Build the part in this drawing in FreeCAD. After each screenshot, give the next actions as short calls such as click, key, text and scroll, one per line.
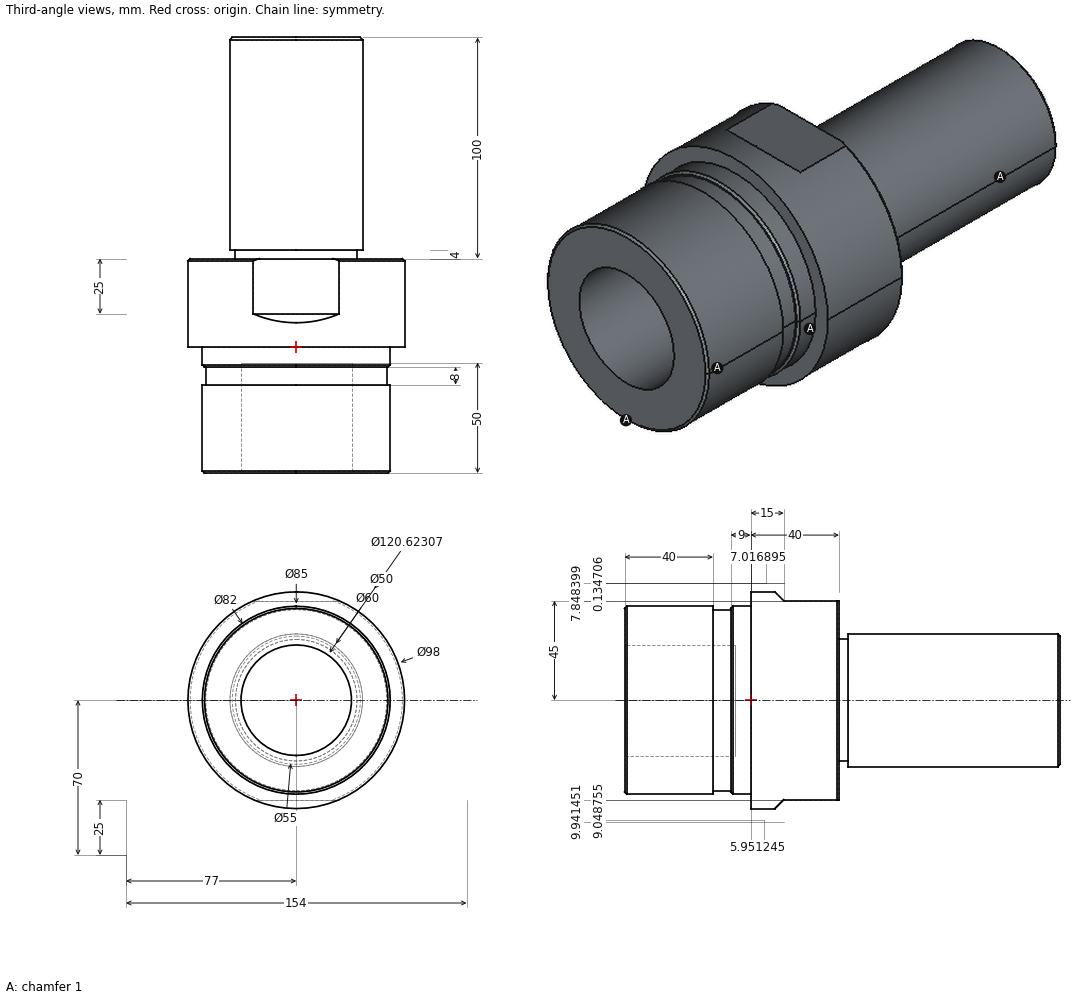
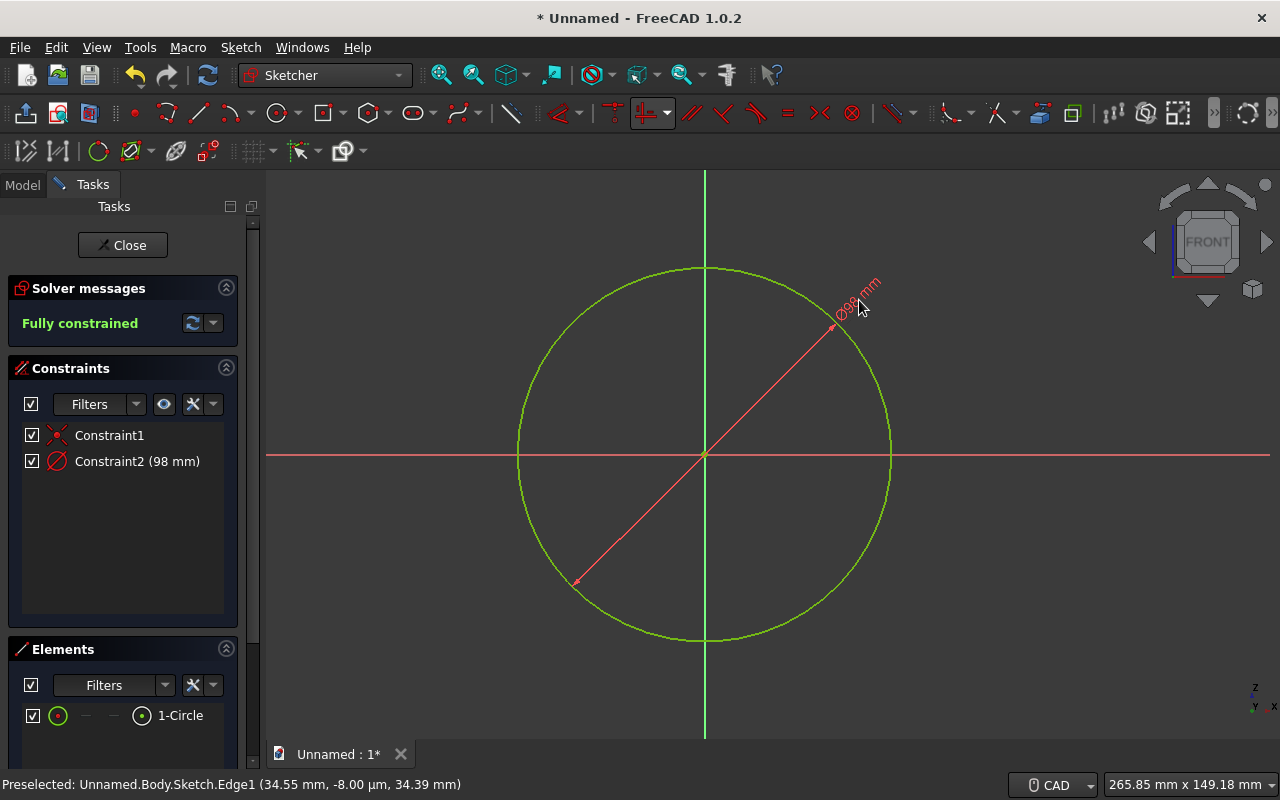
click(123, 245)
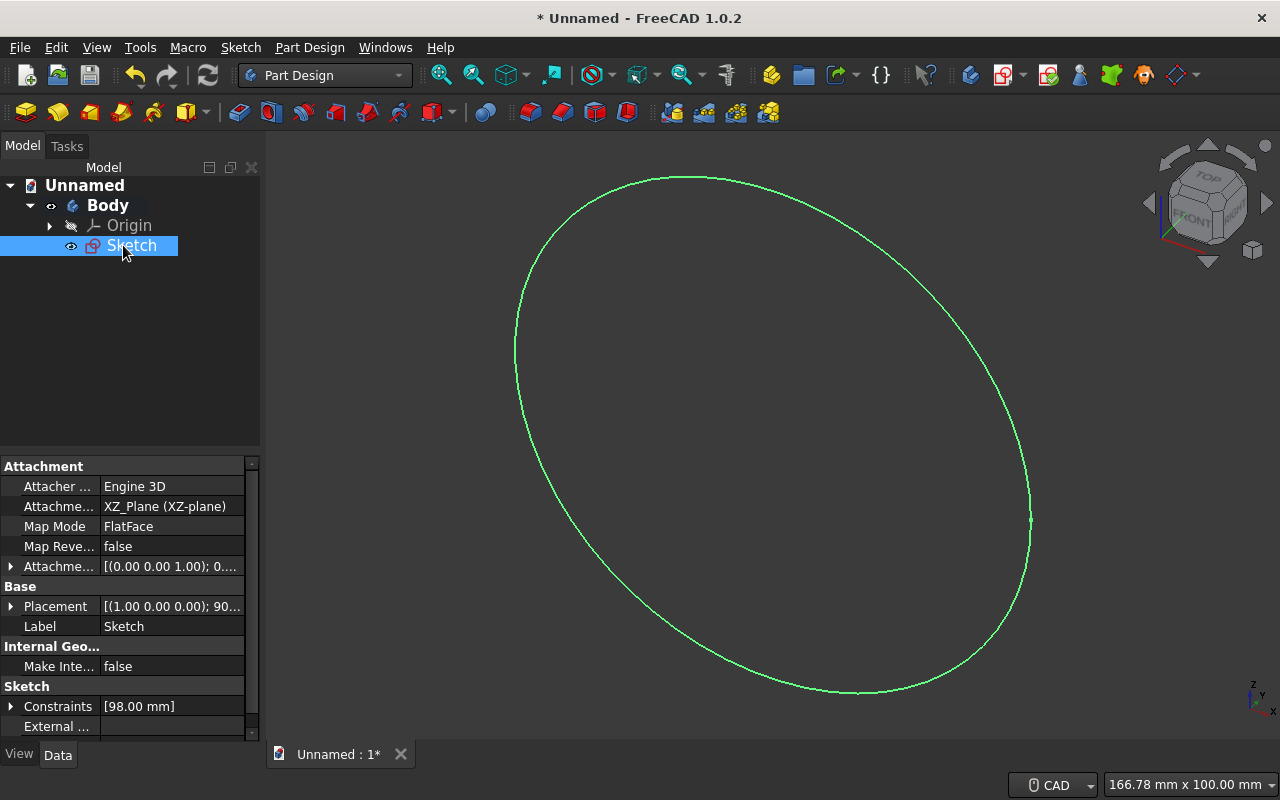
click(26, 112)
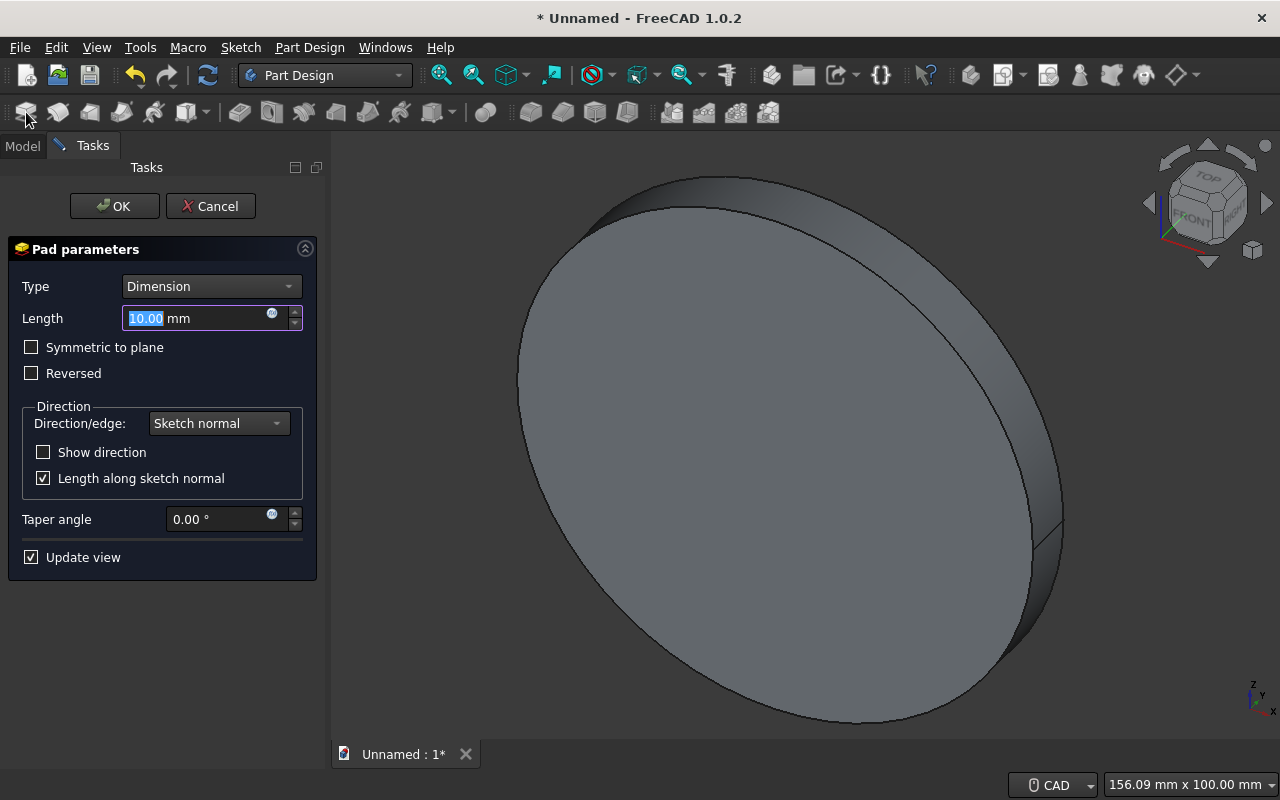
text(40)
key(Tab)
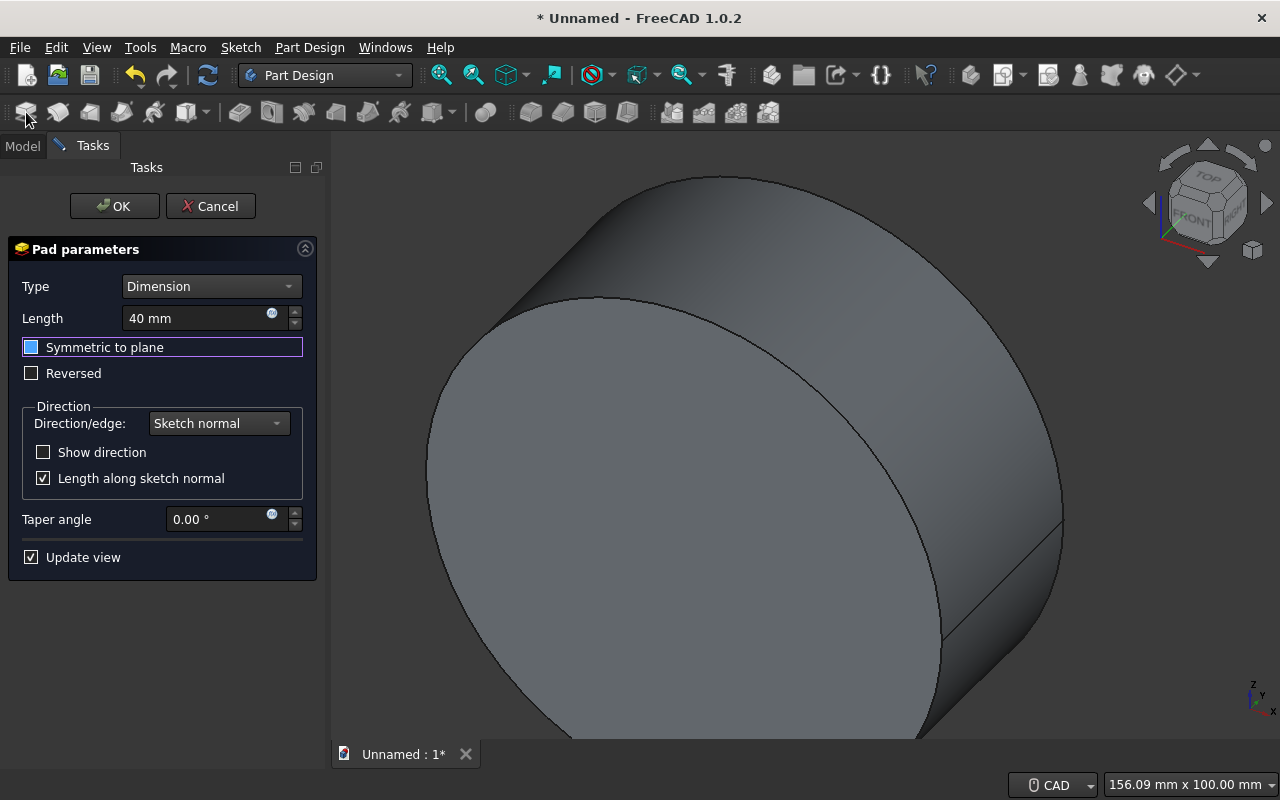
click(30, 373)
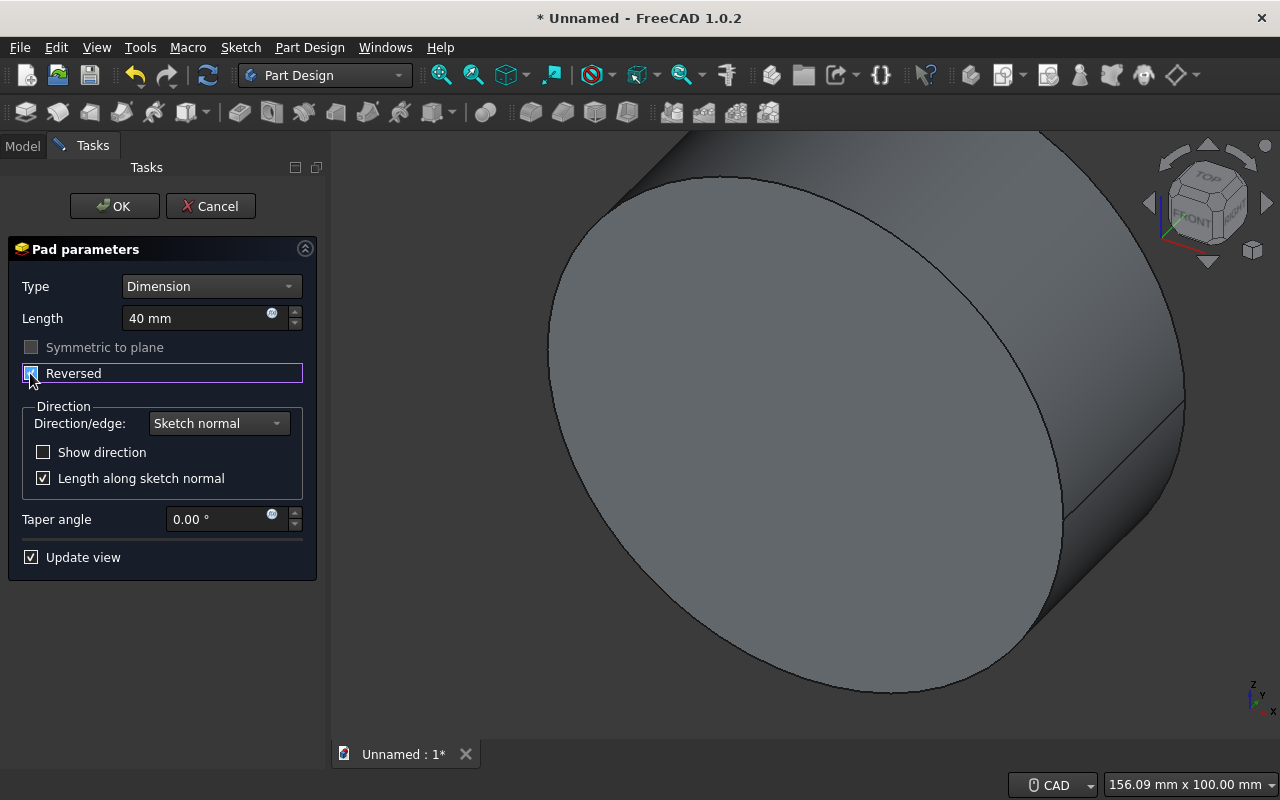
click(115, 206)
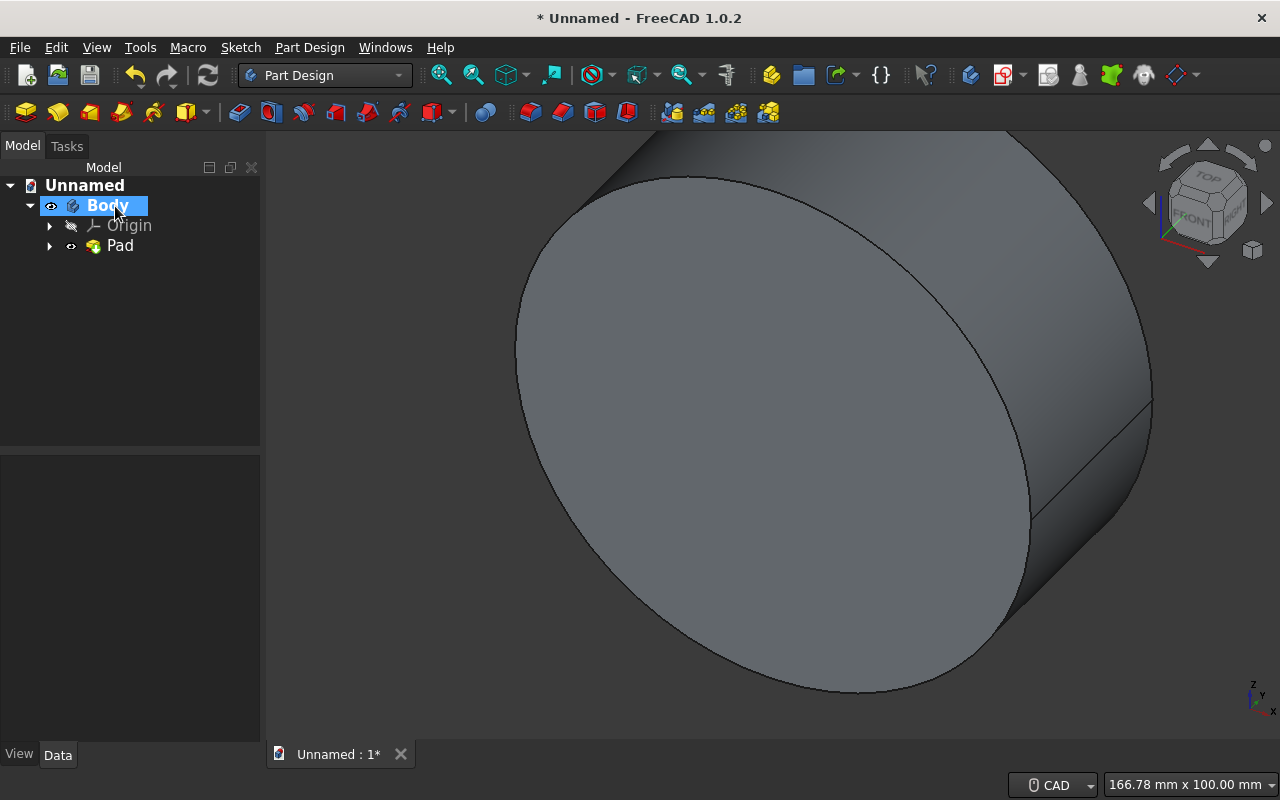
click(442, 76)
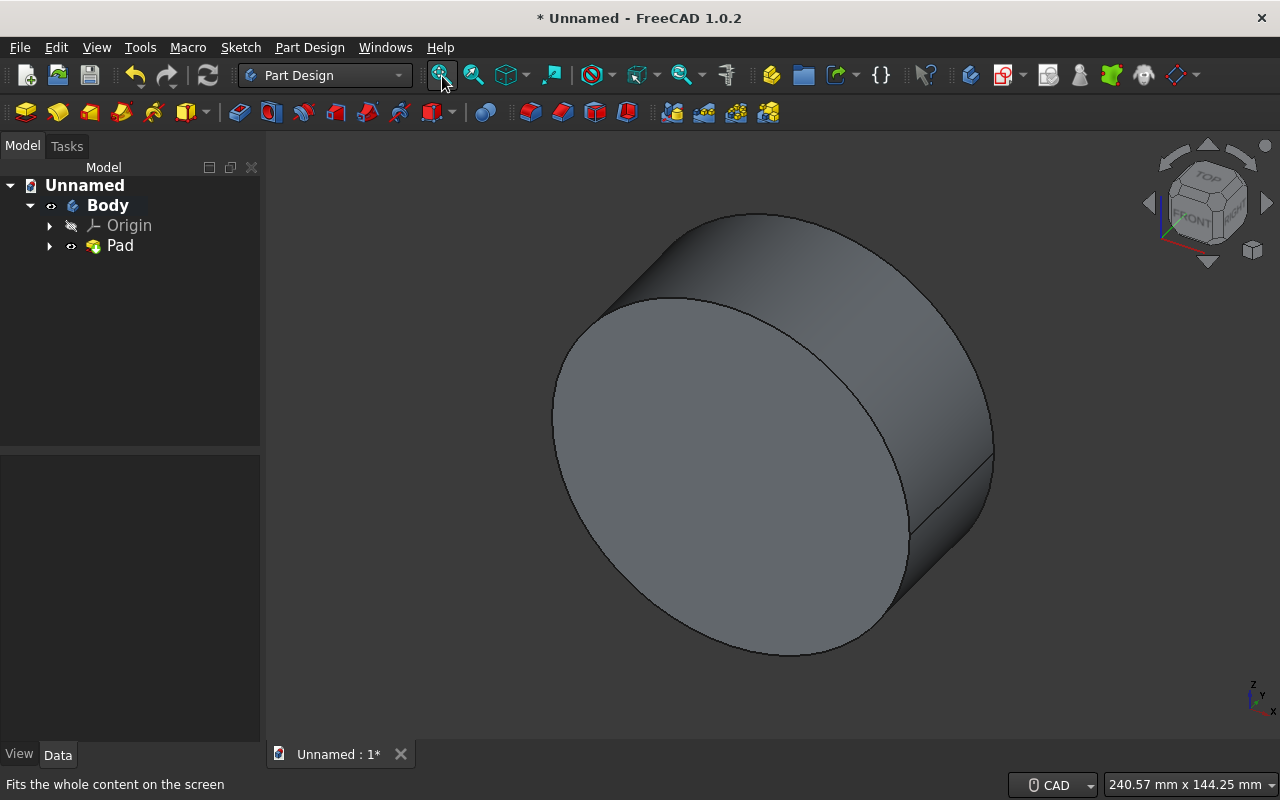
key(4)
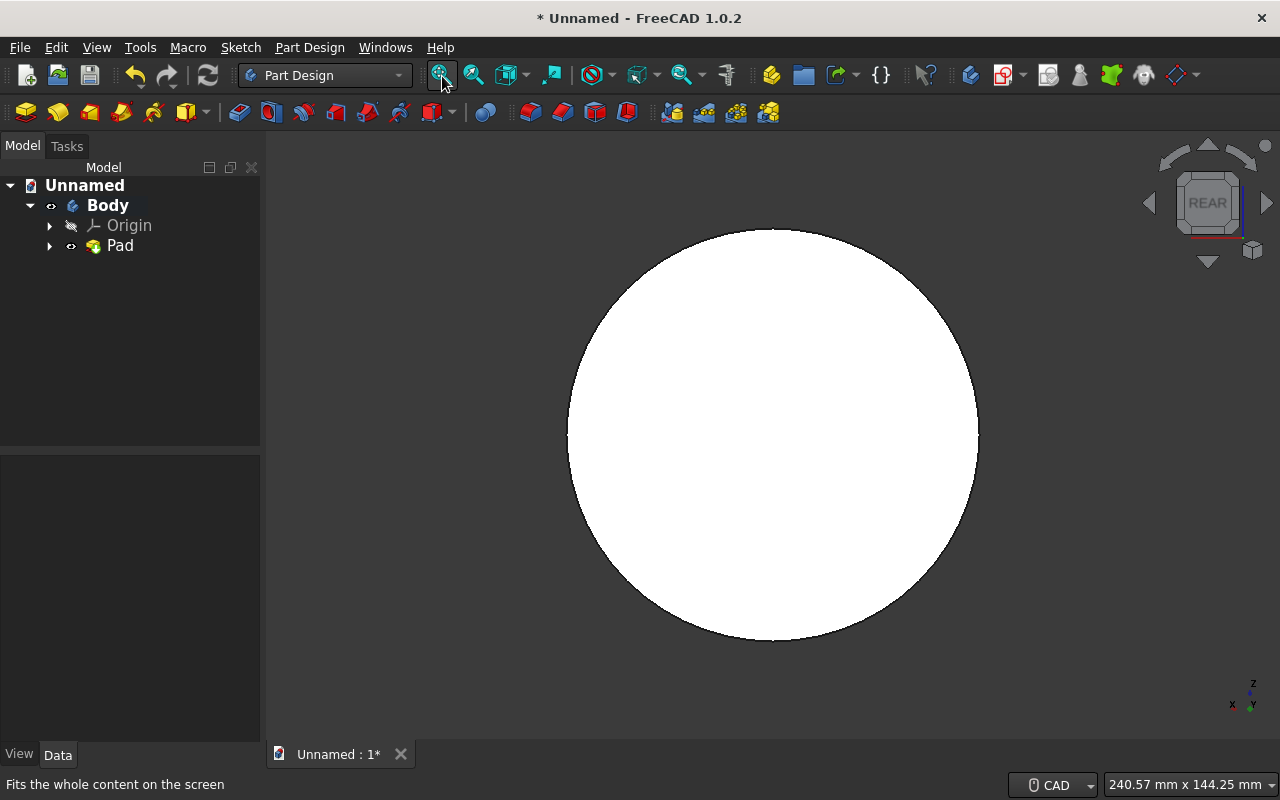
click(773, 434)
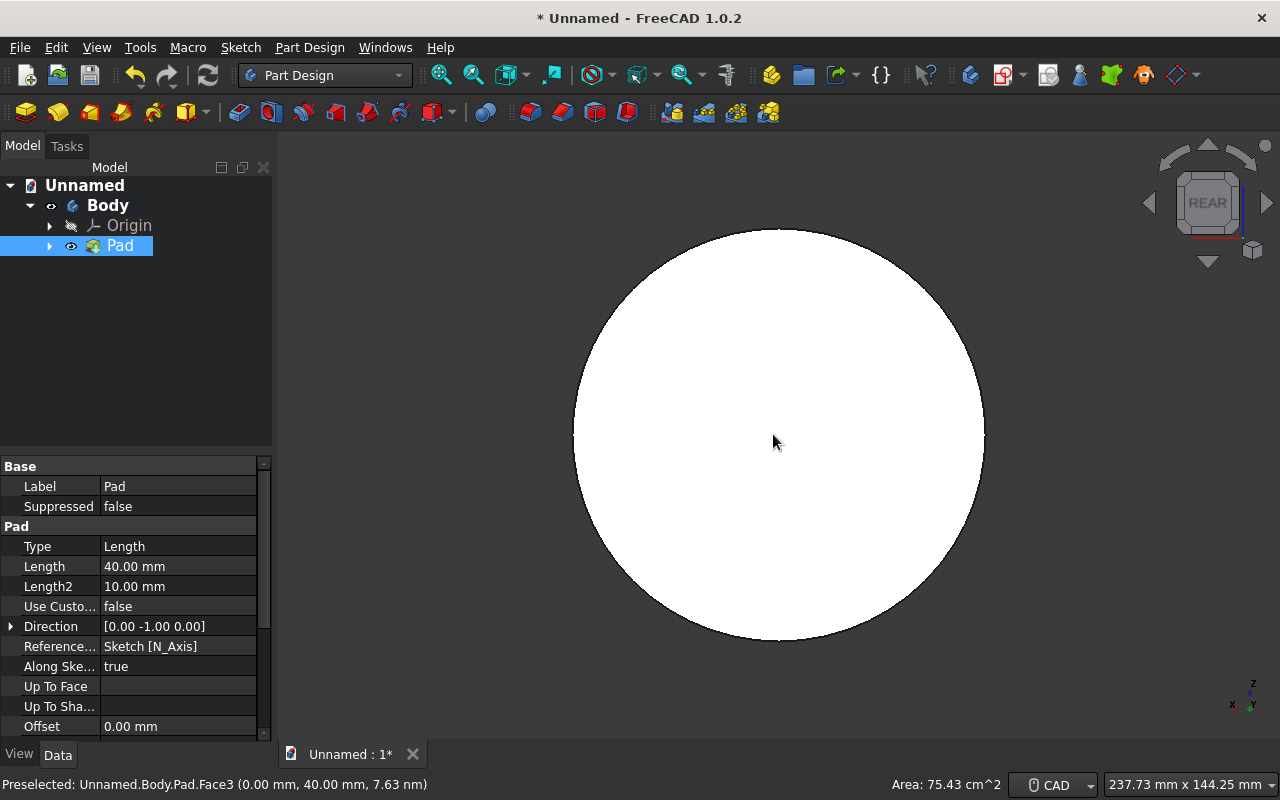
click(1004, 76)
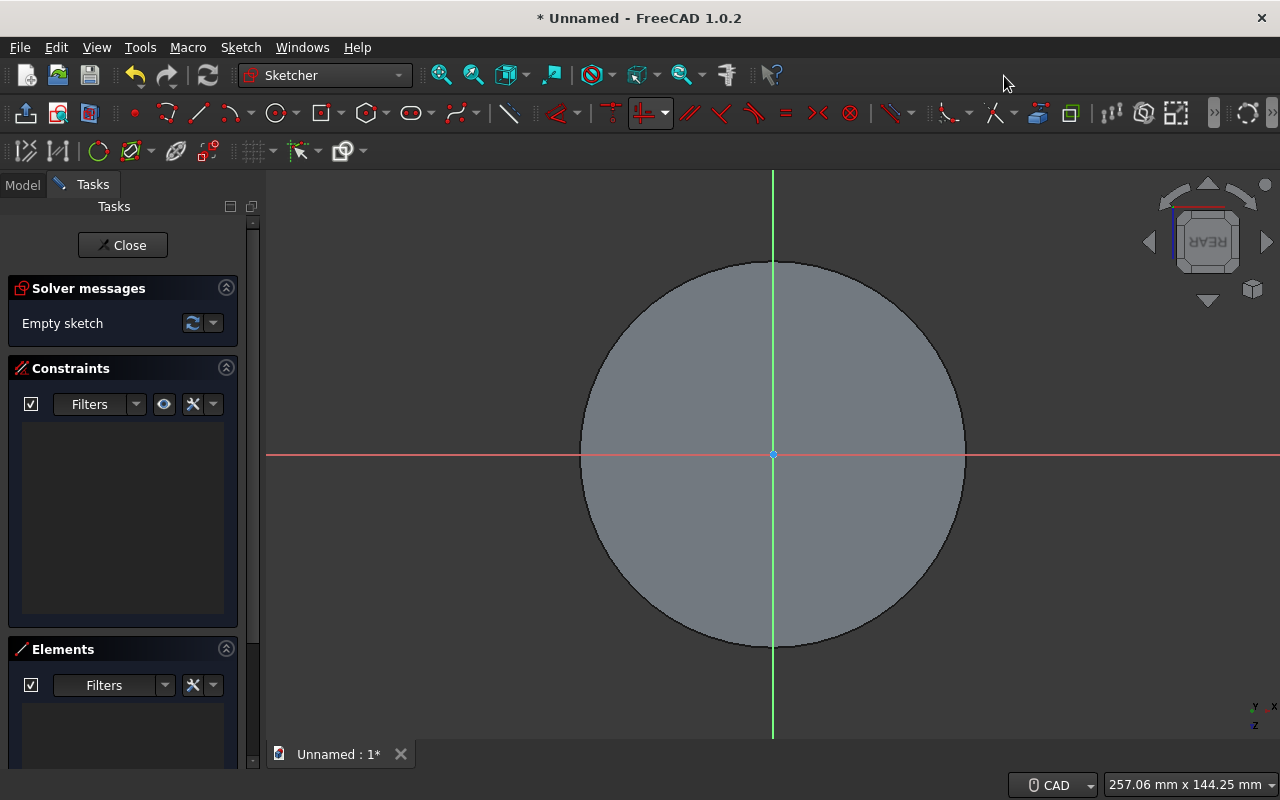
scroll(912, 454, up, 2)